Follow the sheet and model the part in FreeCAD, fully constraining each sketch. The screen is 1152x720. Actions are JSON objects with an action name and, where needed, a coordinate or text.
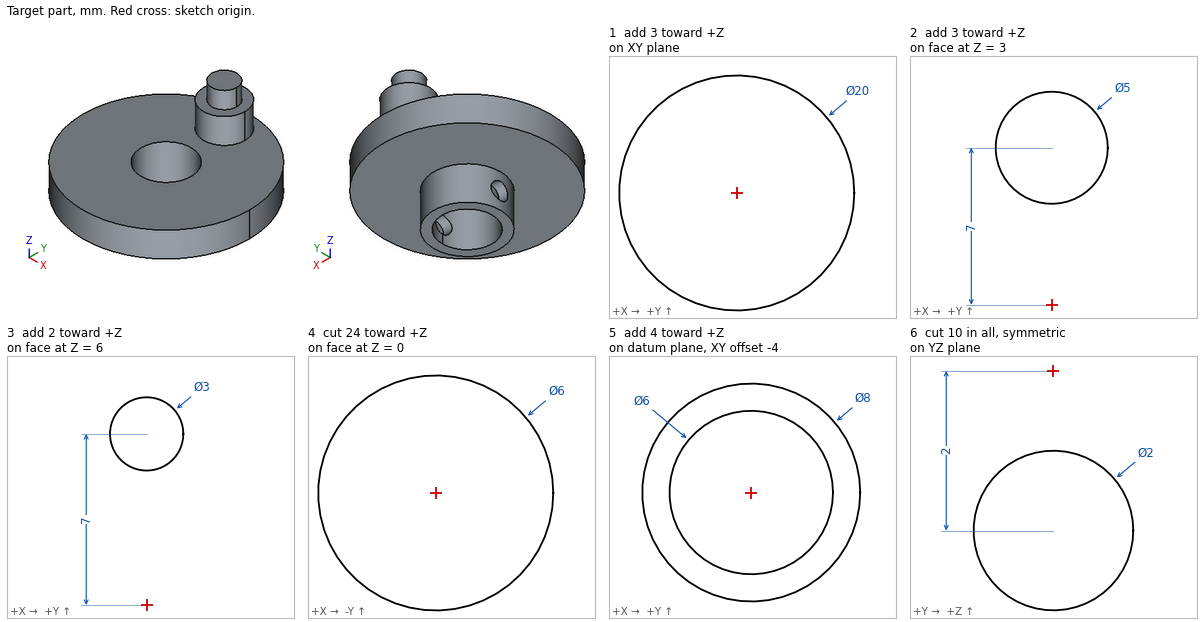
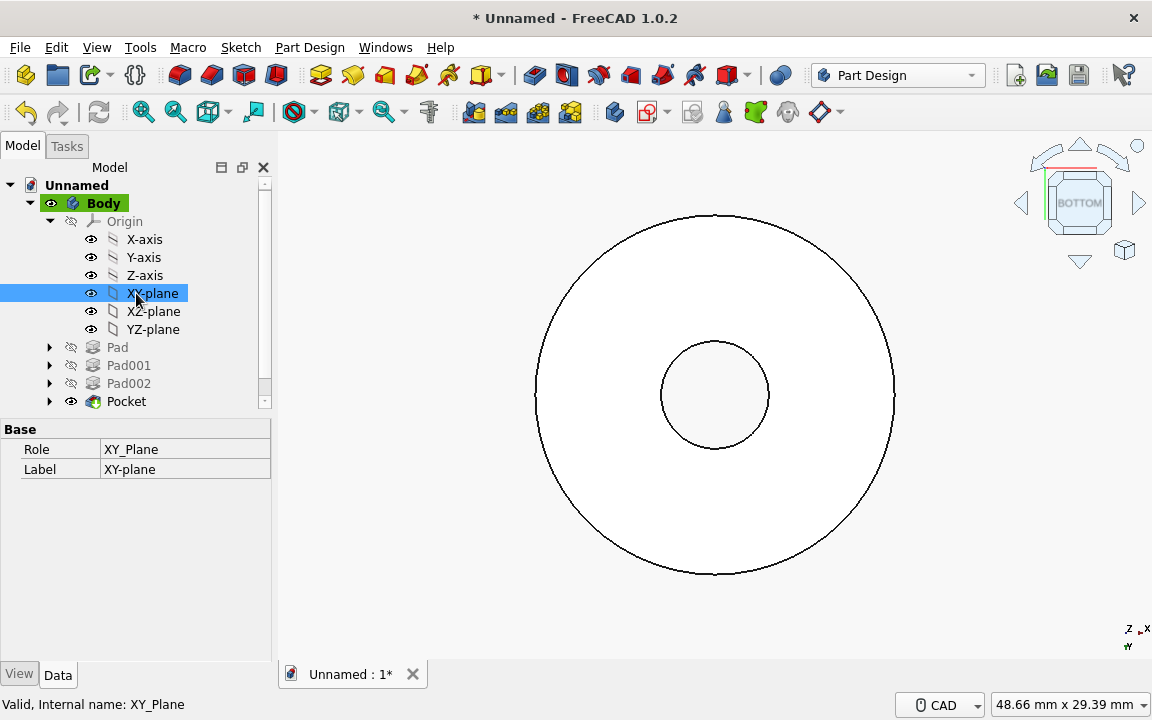
{"action": "left_click", "coordinate": [820, 112]}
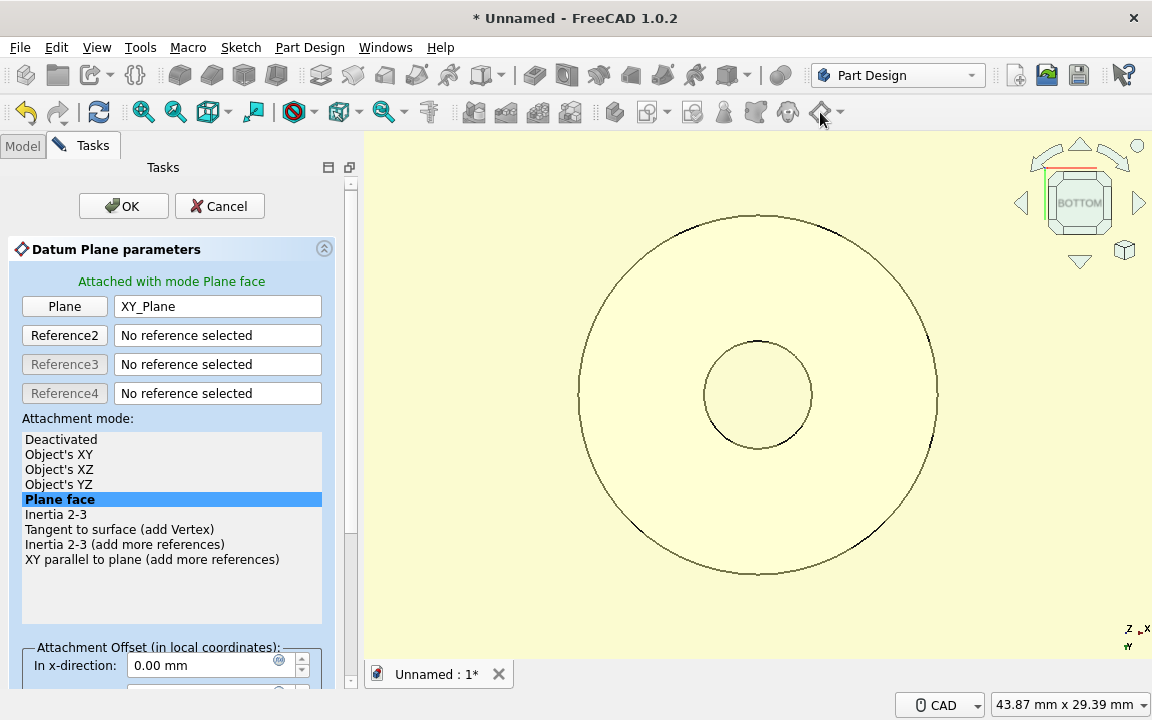
{"action": "scroll", "coordinate": [351, 432], "scroll_direction": "down", "scroll_amount": 2}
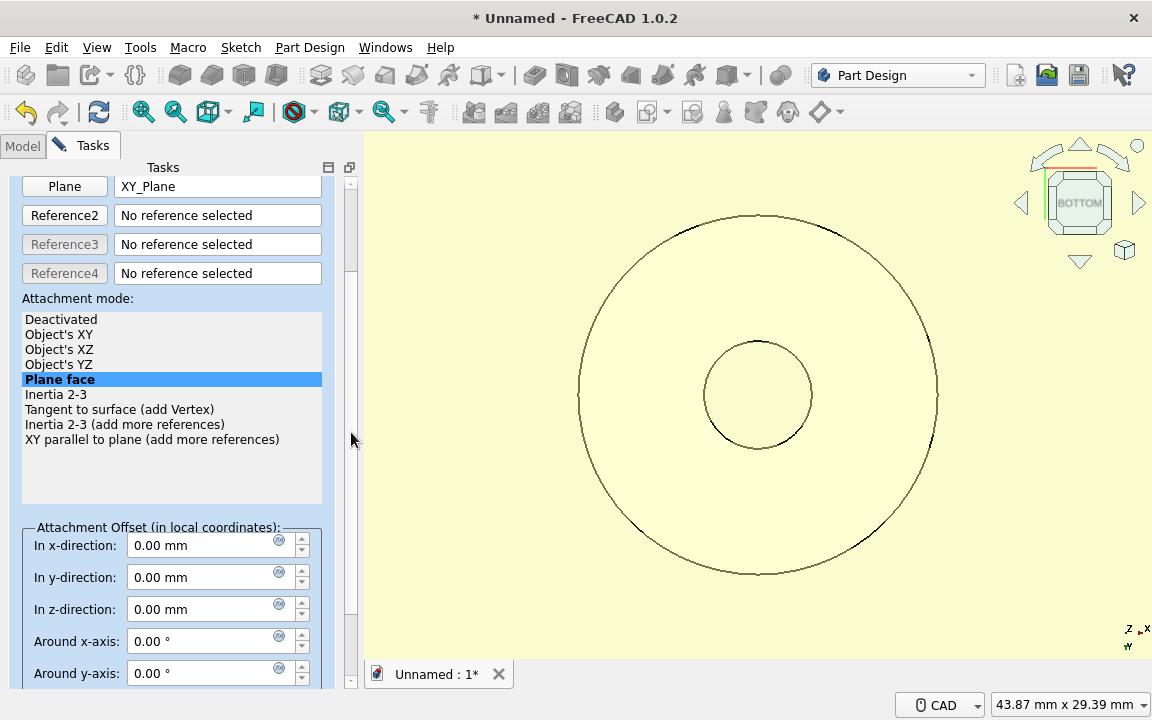
{"action": "triple_click", "coordinate": [210, 609]}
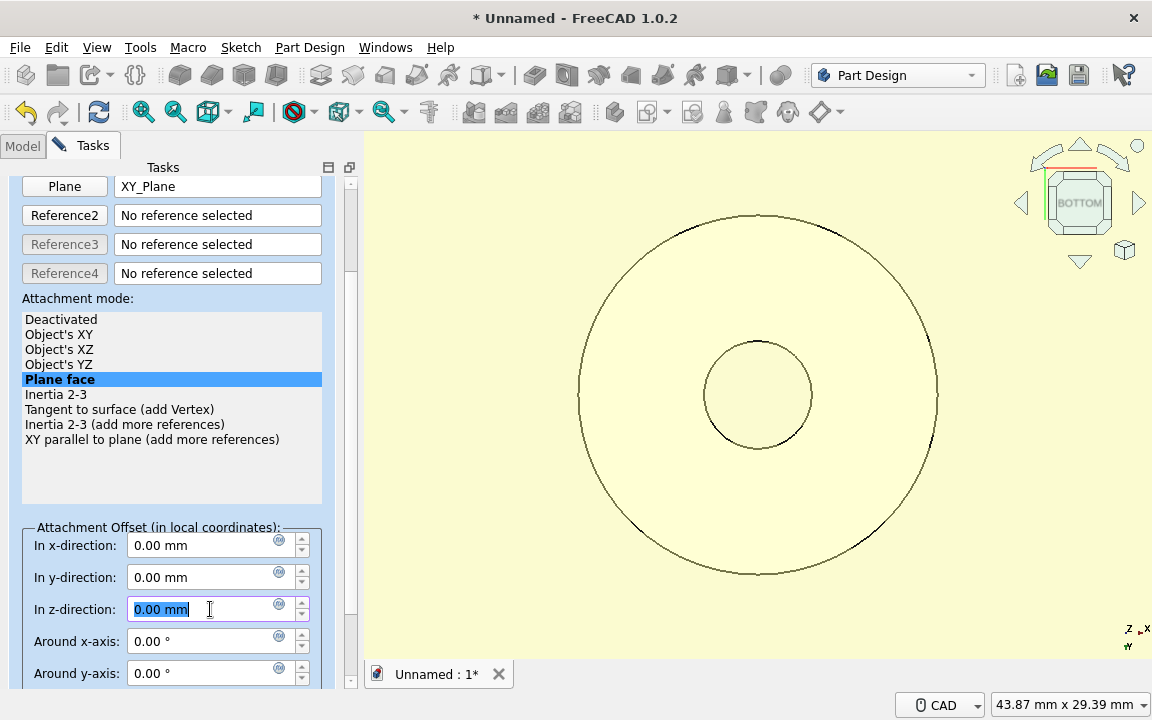
{"action": "type", "text": "-4"}
{"action": "key", "text": "Tab"}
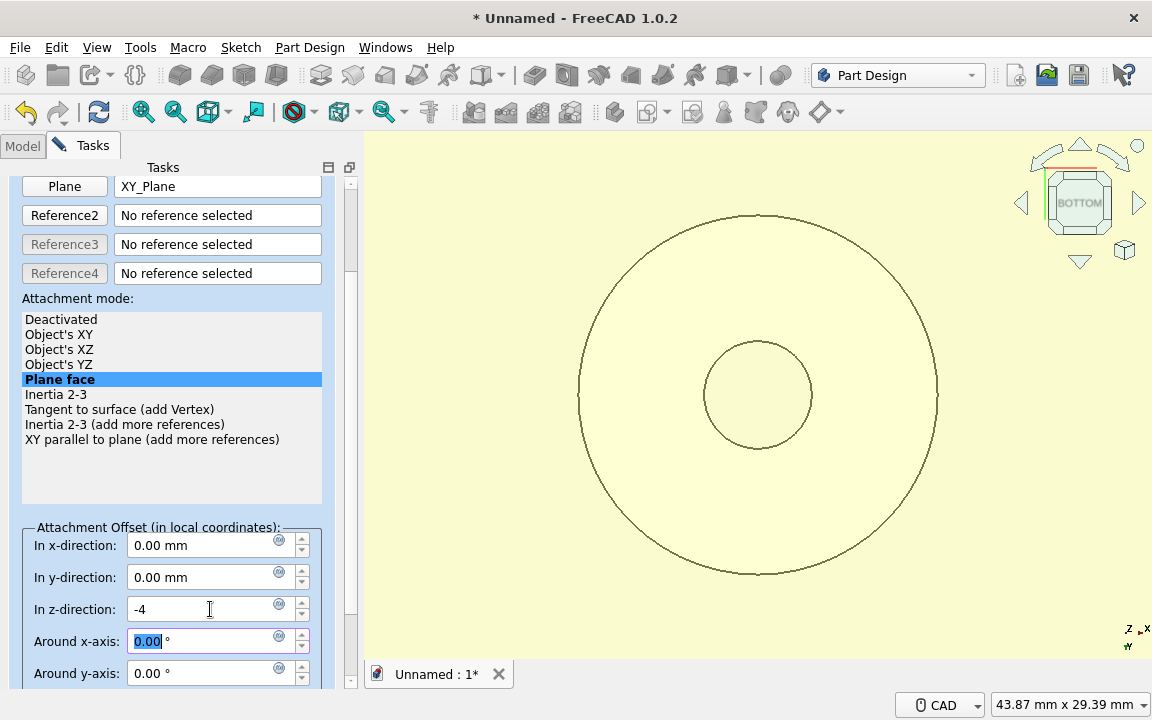
{"action": "scroll", "coordinate": [351, 432], "scroll_direction": "up", "scroll_amount": 3}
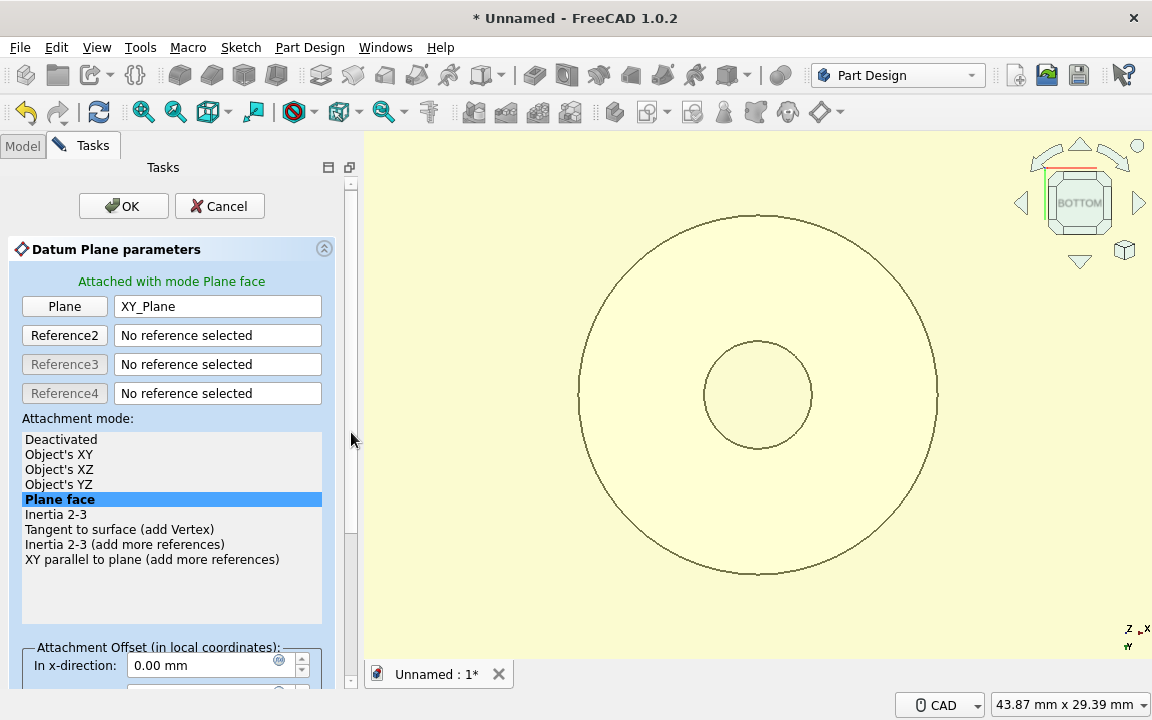
{"action": "left_click", "coordinate": [124, 206]}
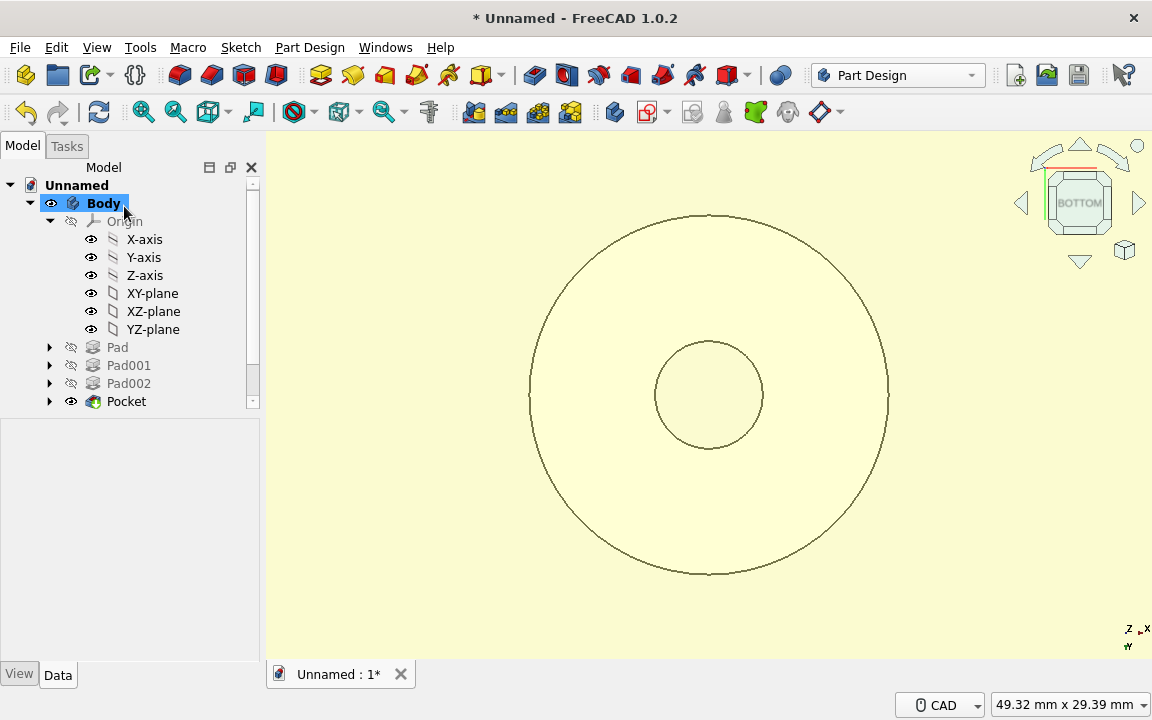
{"action": "scroll", "coordinate": [100, 289], "scroll_direction": "down", "scroll_amount": 3}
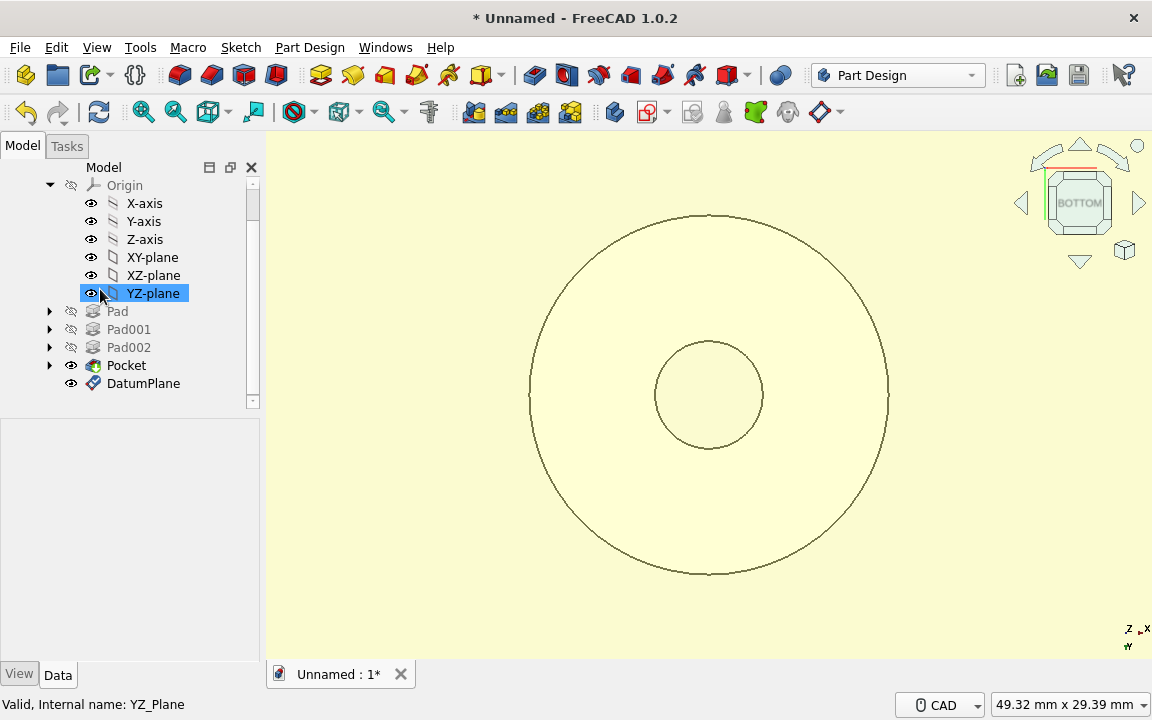
{"action": "left_click", "coordinate": [116, 383]}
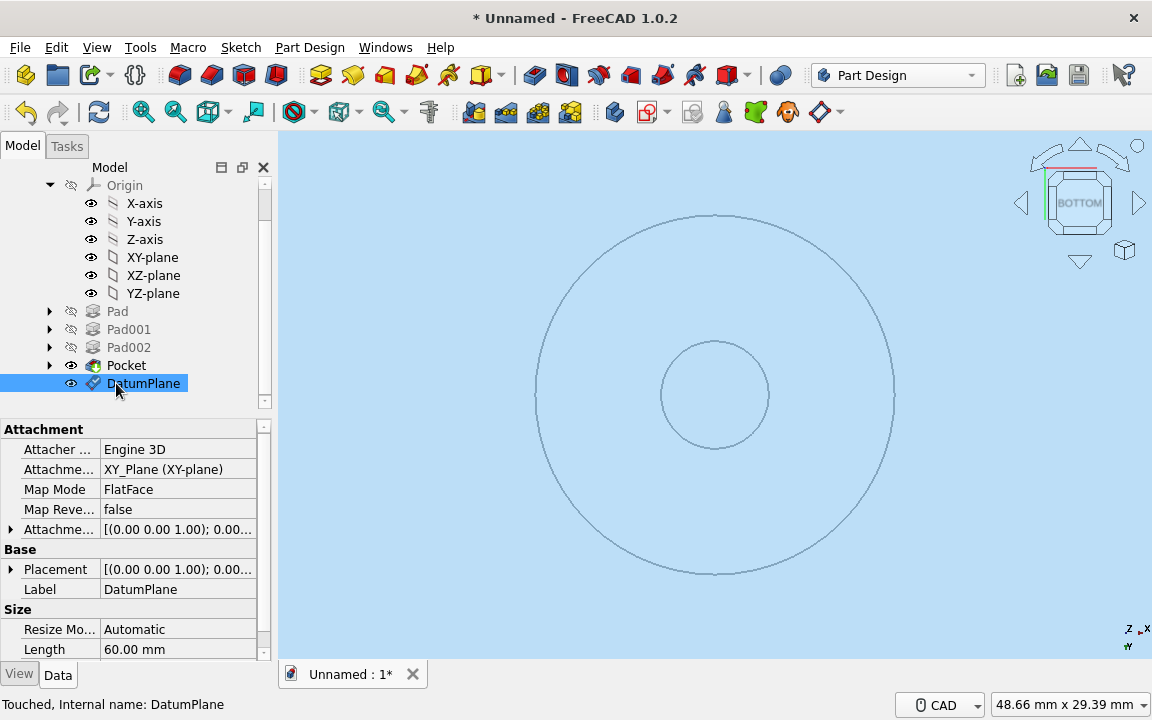
{"action": "left_click", "coordinate": [648, 112]}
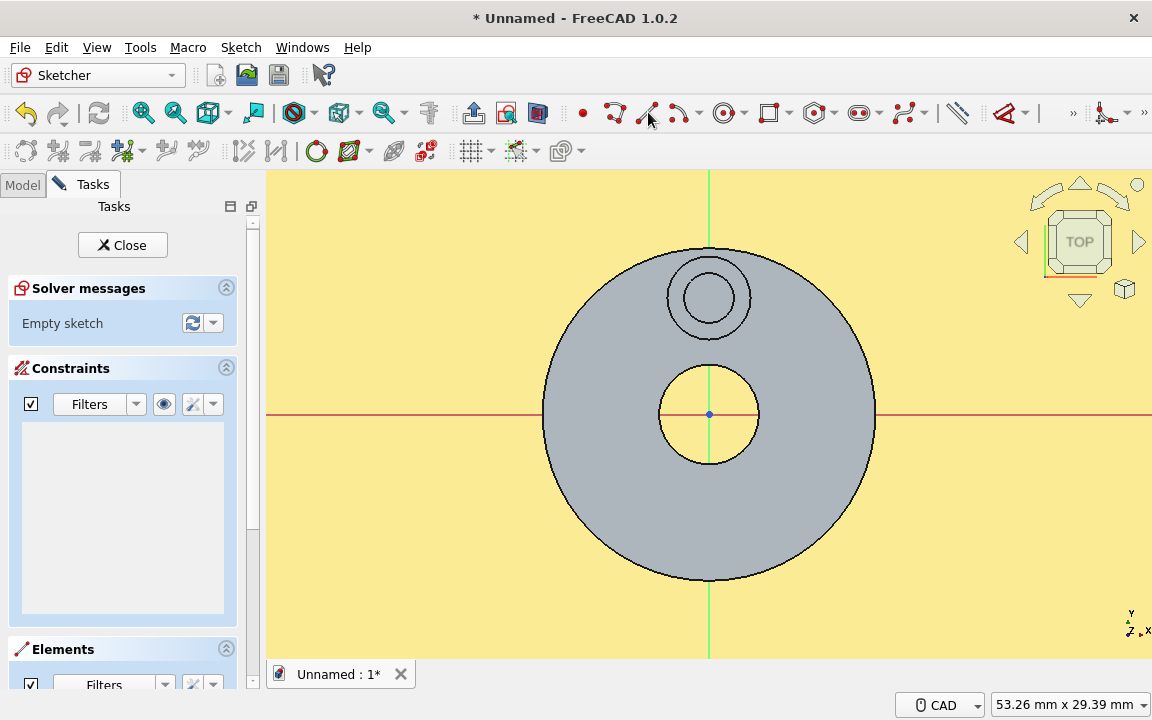
{"action": "key", "text": "q s"}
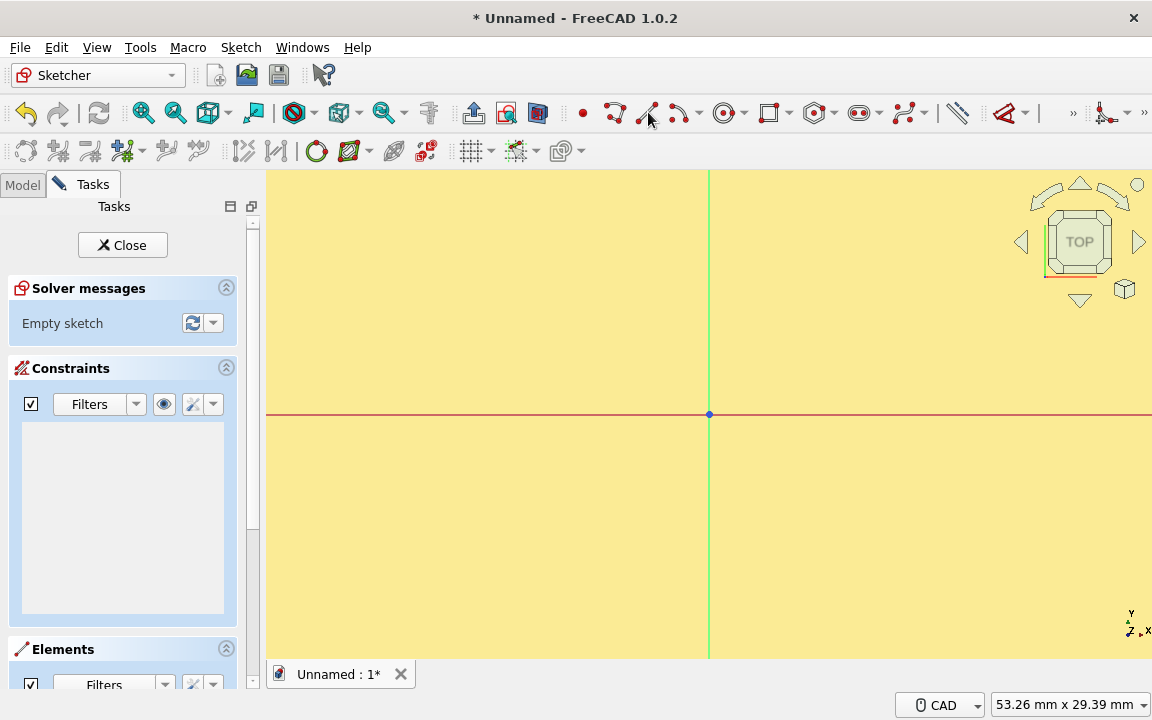
{"action": "scroll", "coordinate": [765, 414], "scroll_direction": "up", "scroll_amount": 4}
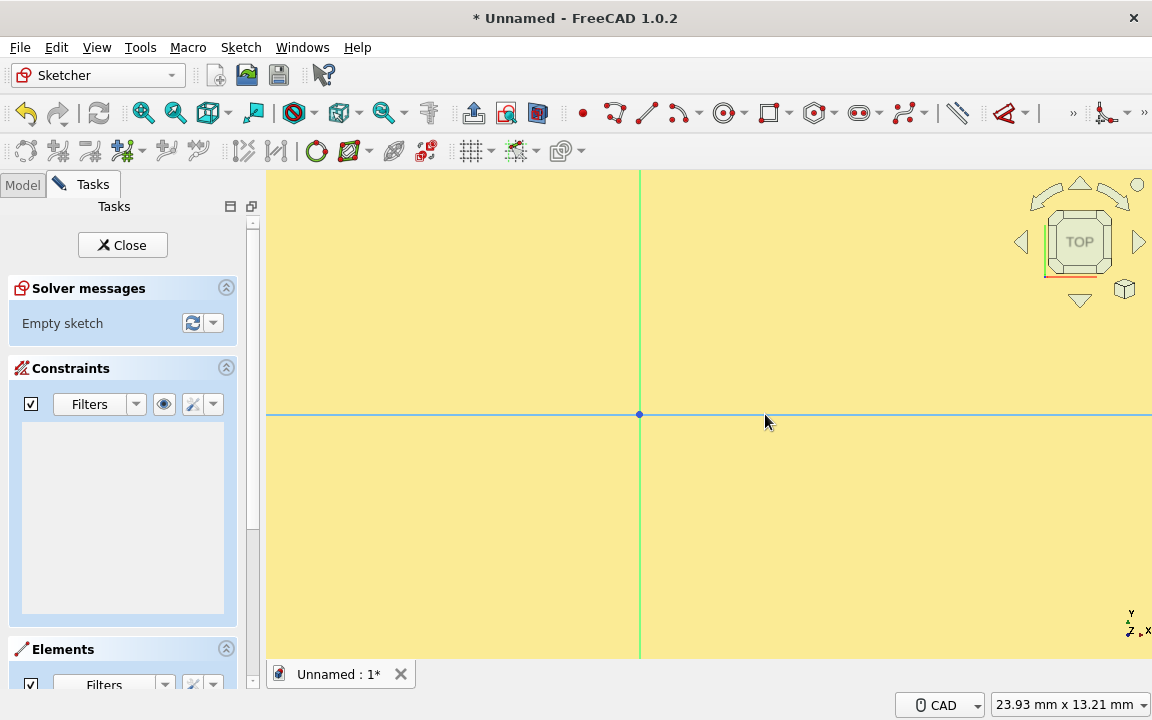
{"action": "left_click", "coordinate": [724, 114]}